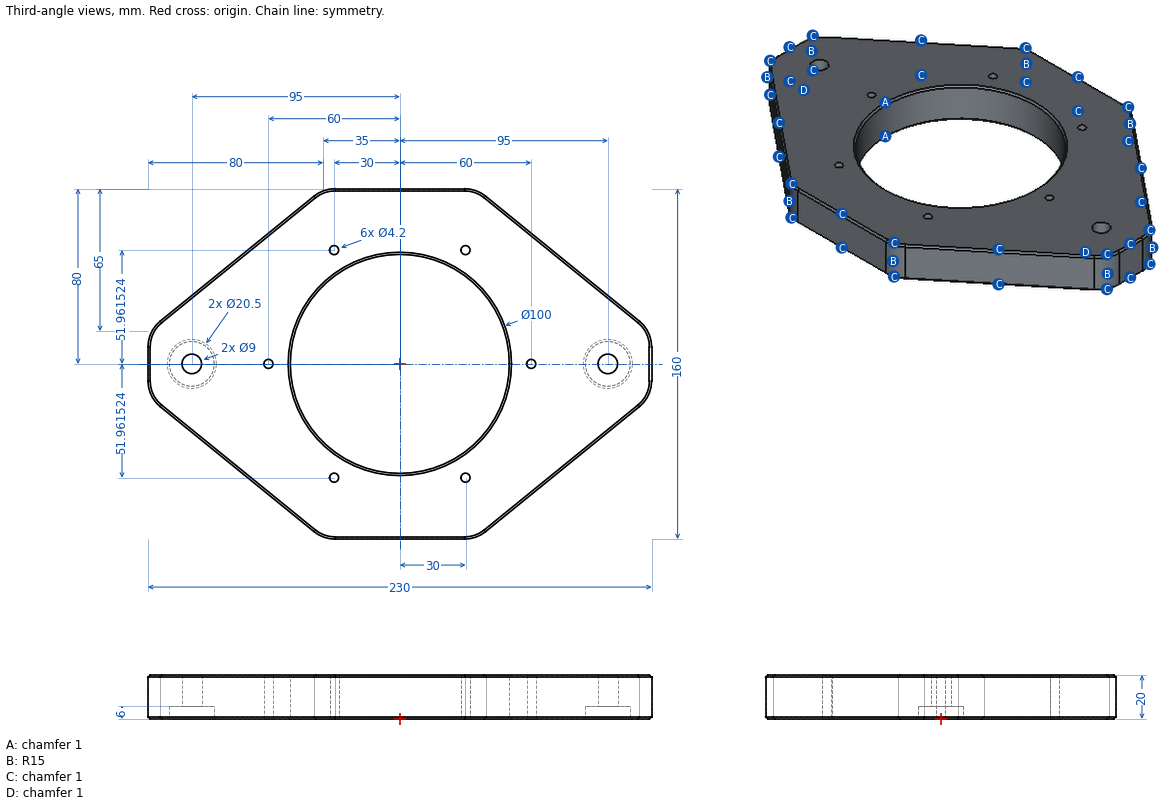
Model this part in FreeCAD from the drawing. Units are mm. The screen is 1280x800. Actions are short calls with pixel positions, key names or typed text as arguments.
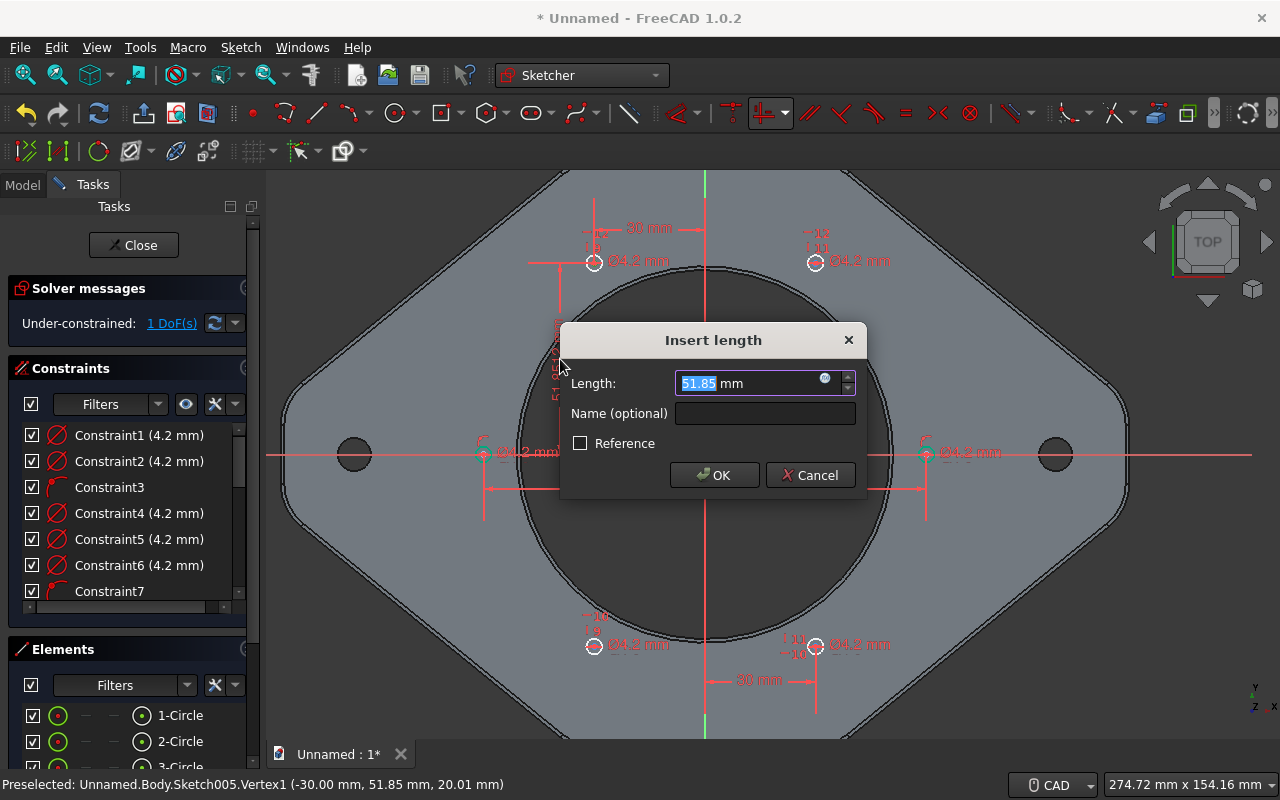
text(51.961524)
key(Return)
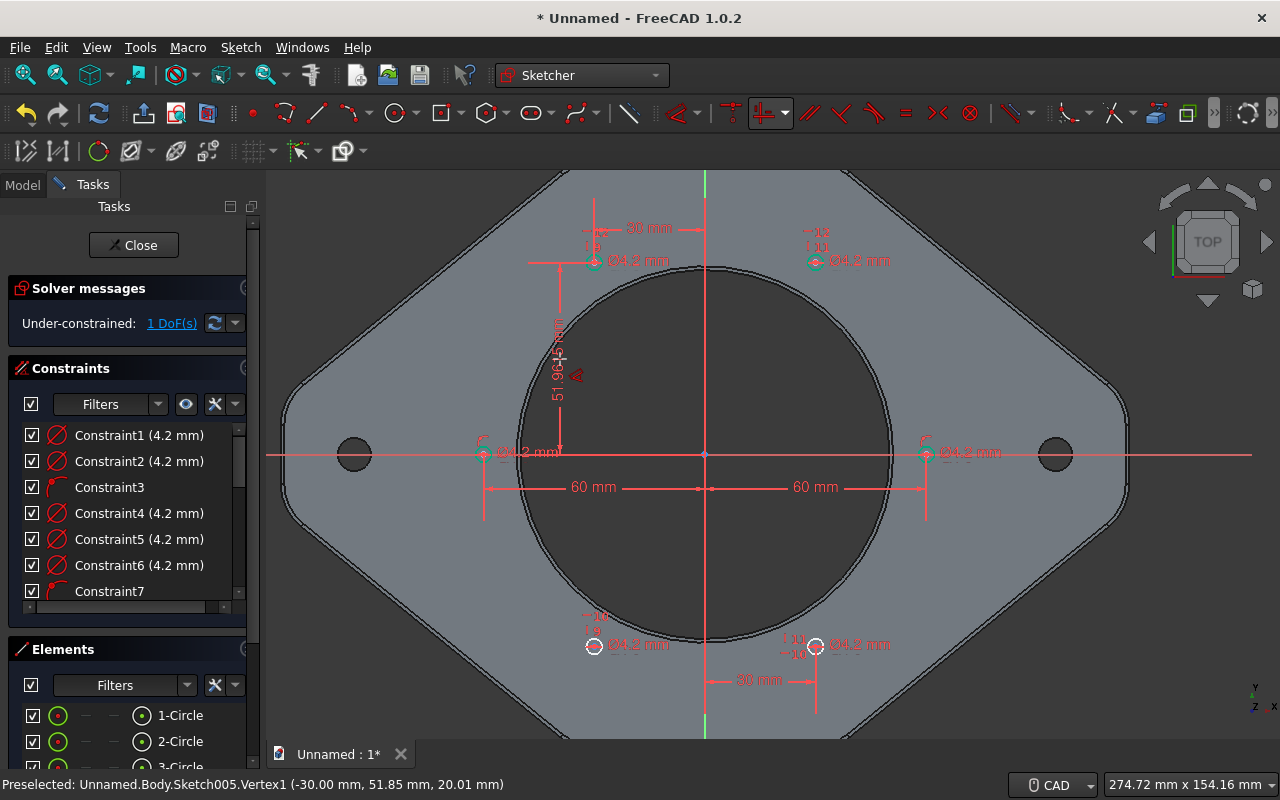
click(594, 647)
click(560, 551)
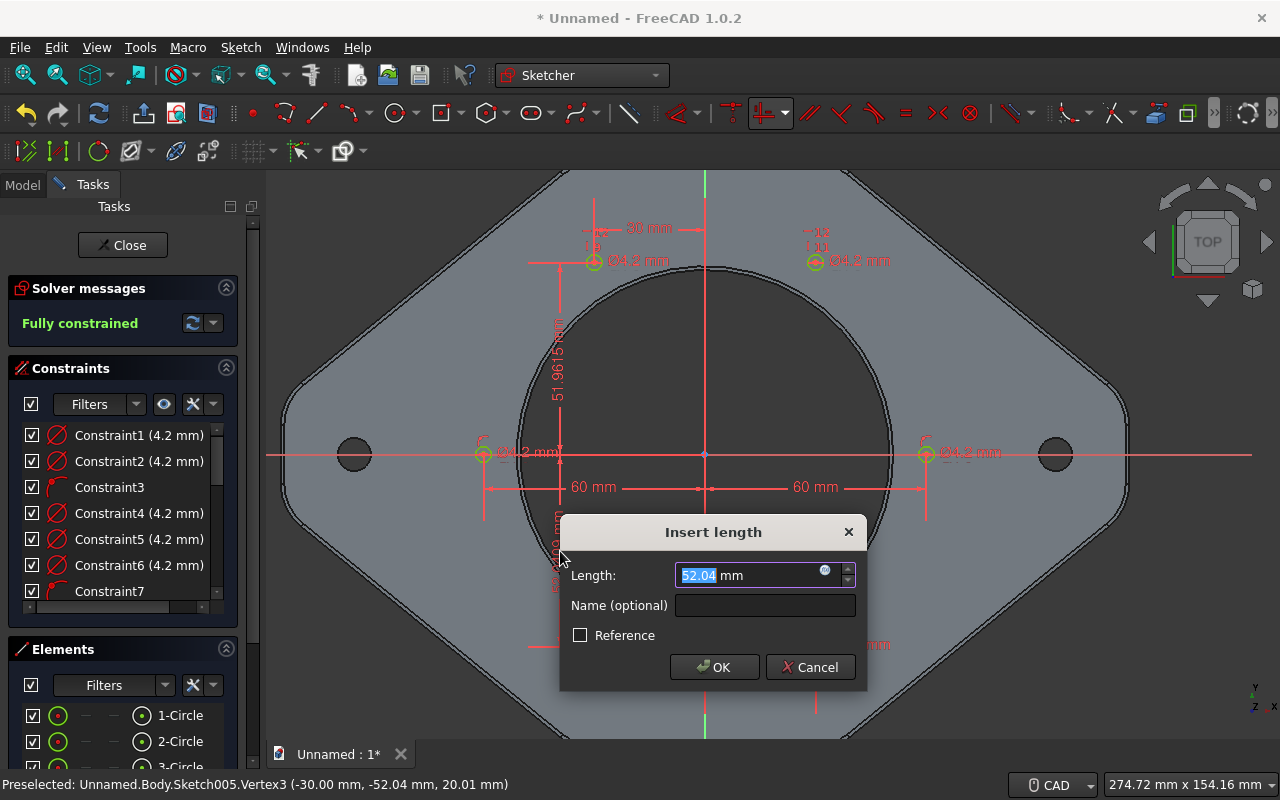
text(51.961524)
key(Return)
key(Escape)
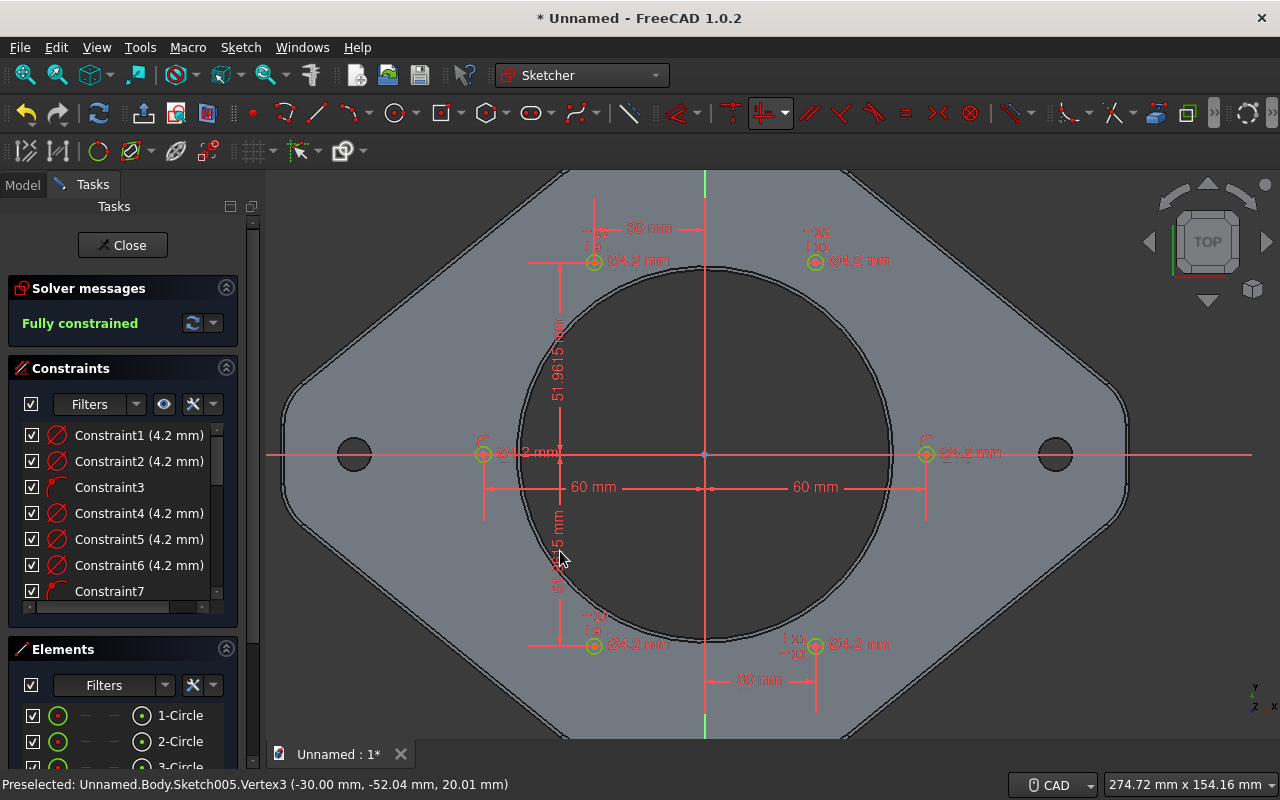
click(123, 245)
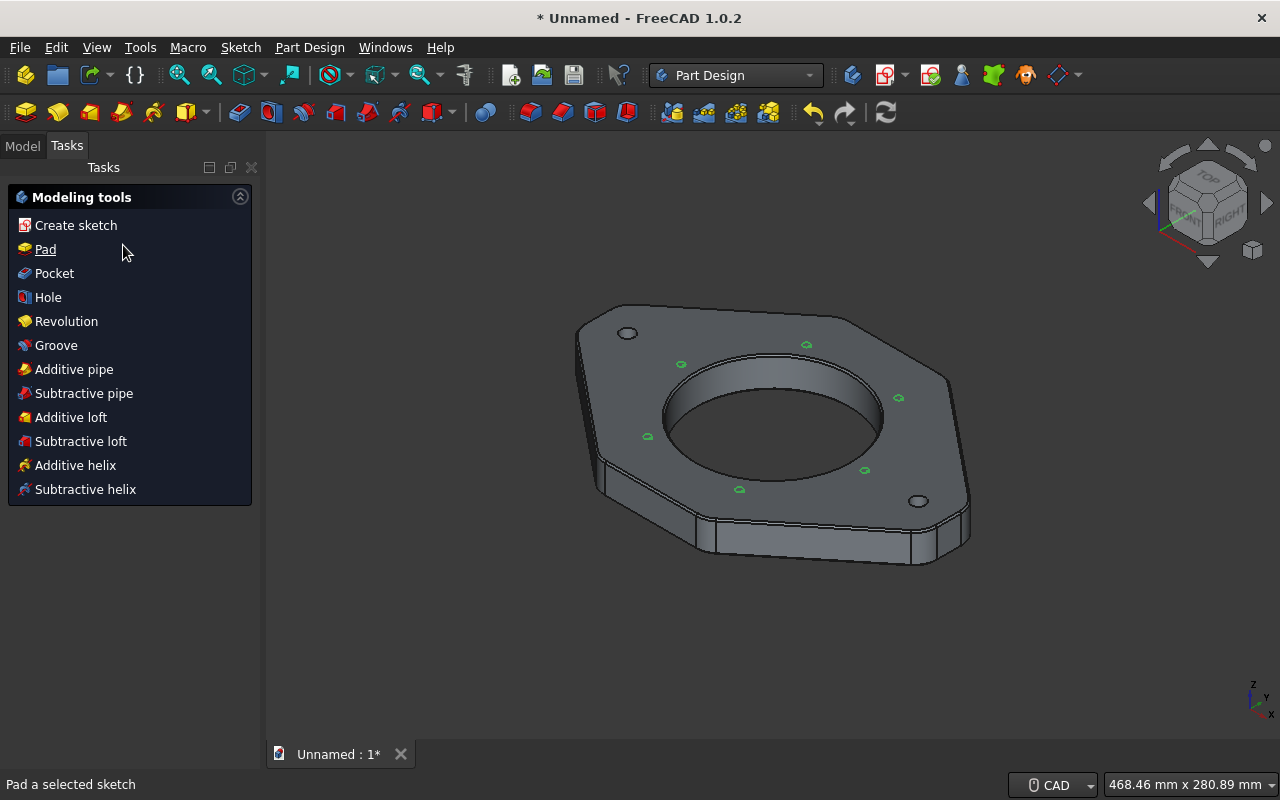
click(240, 112)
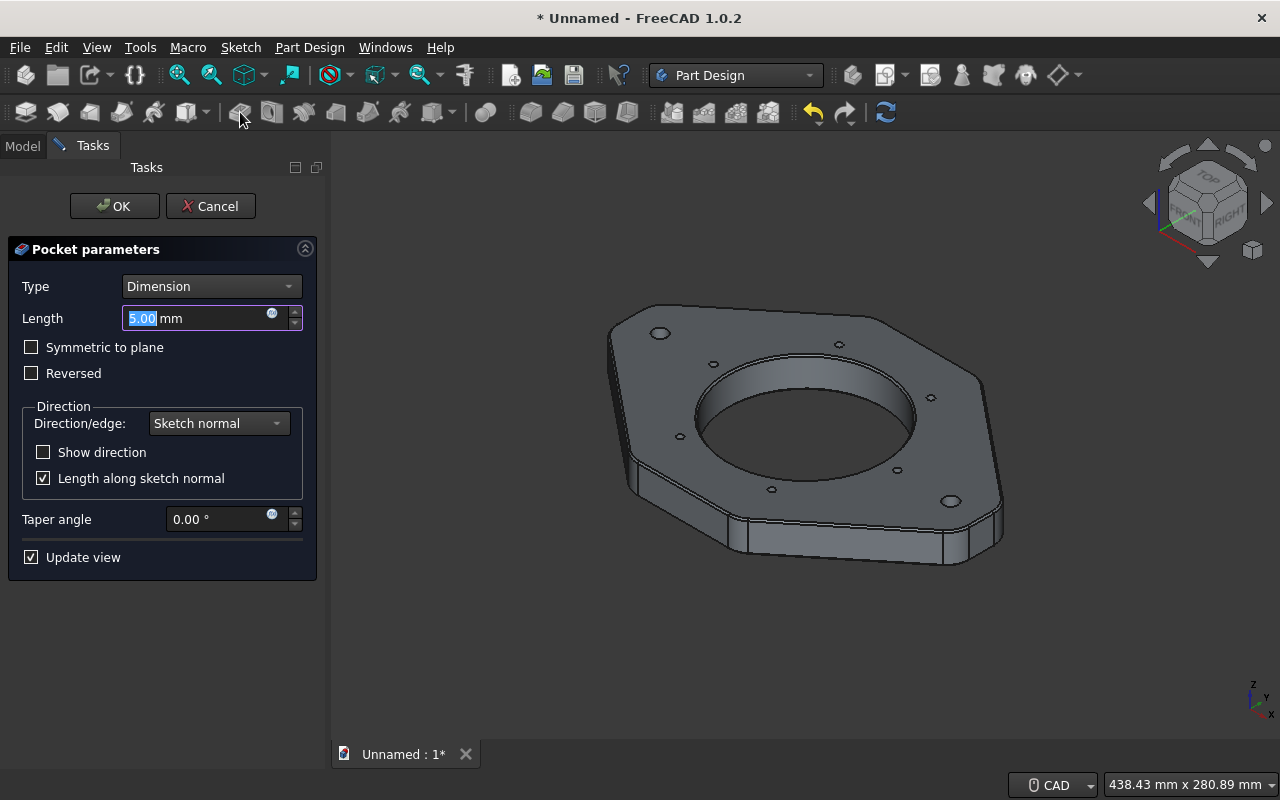
click(212, 286)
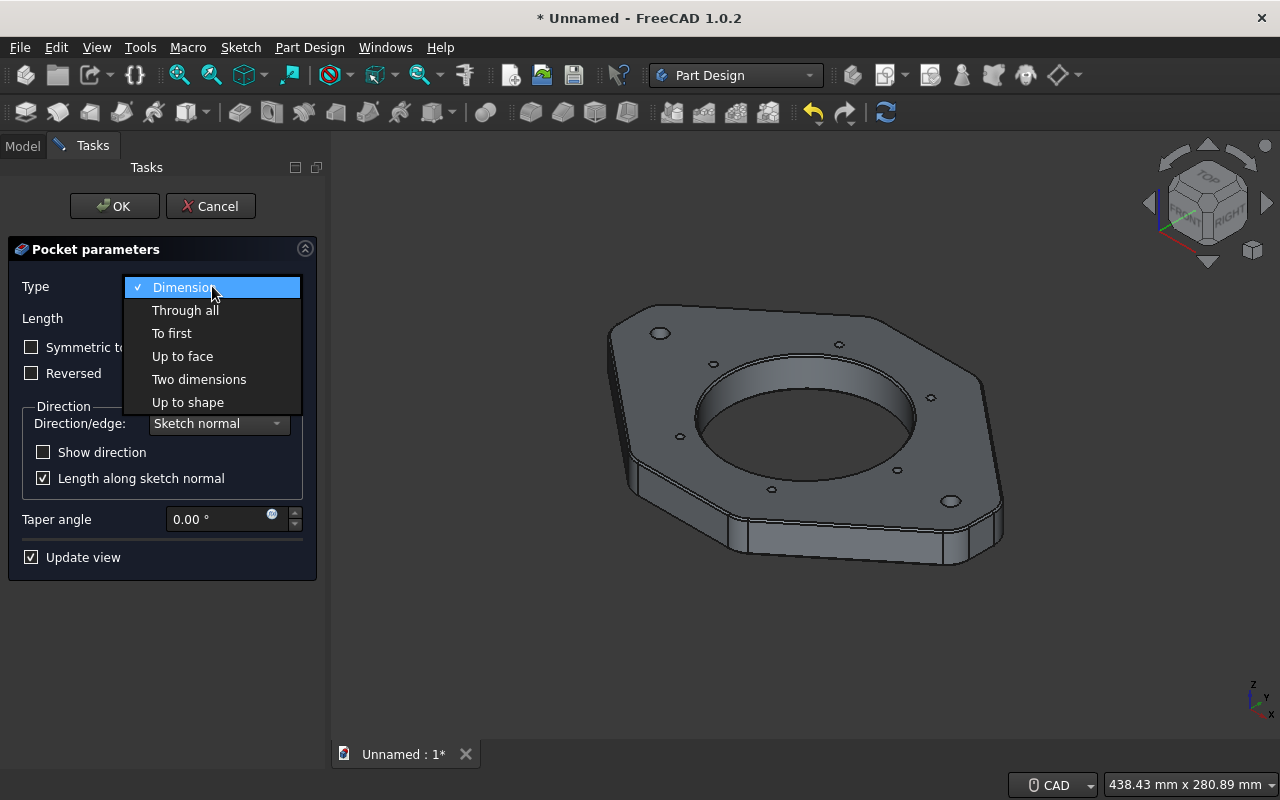
click(212, 310)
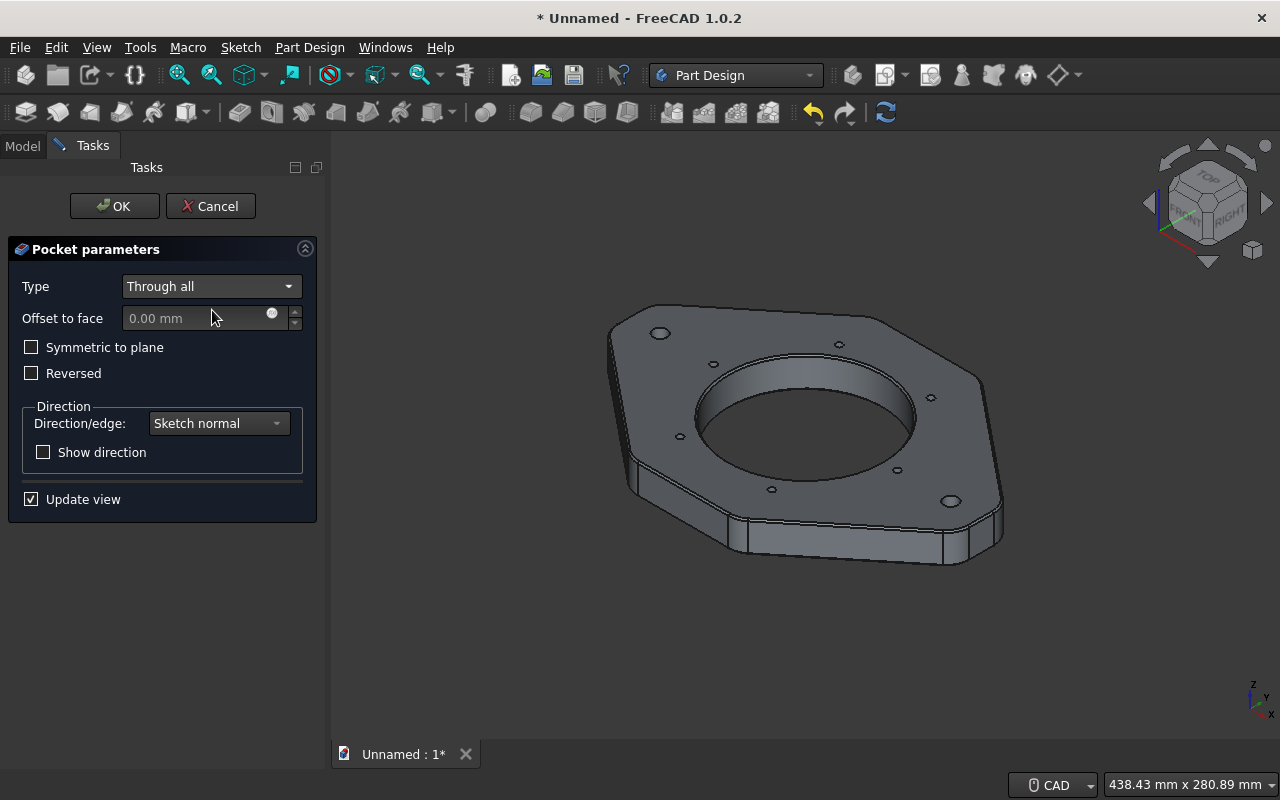
click(115, 206)